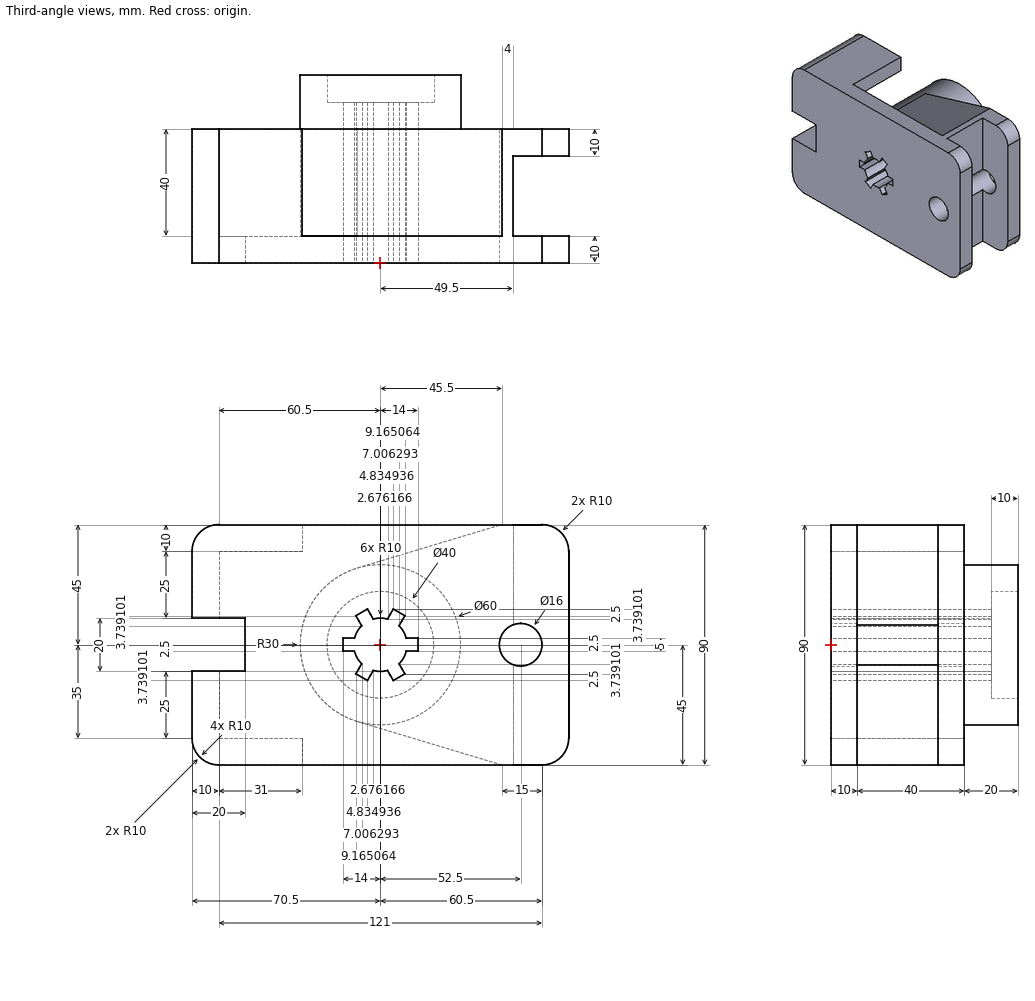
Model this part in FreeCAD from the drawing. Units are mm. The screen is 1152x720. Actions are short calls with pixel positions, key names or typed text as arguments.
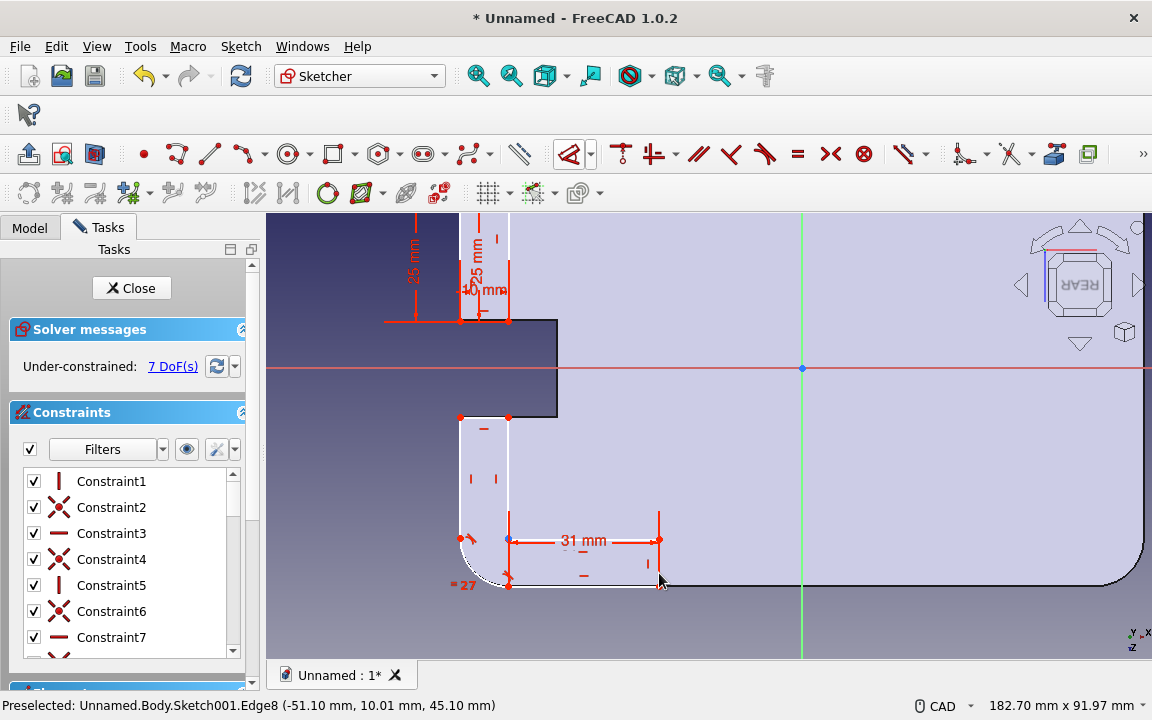
click(659, 573)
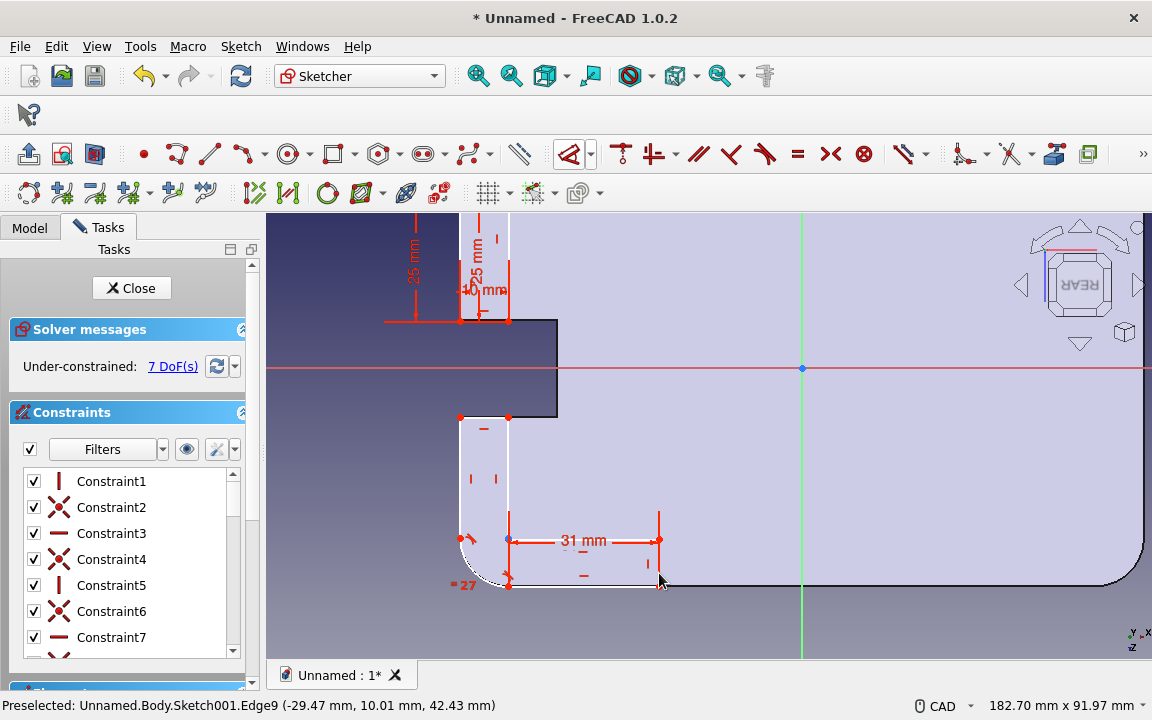
click(590, 154)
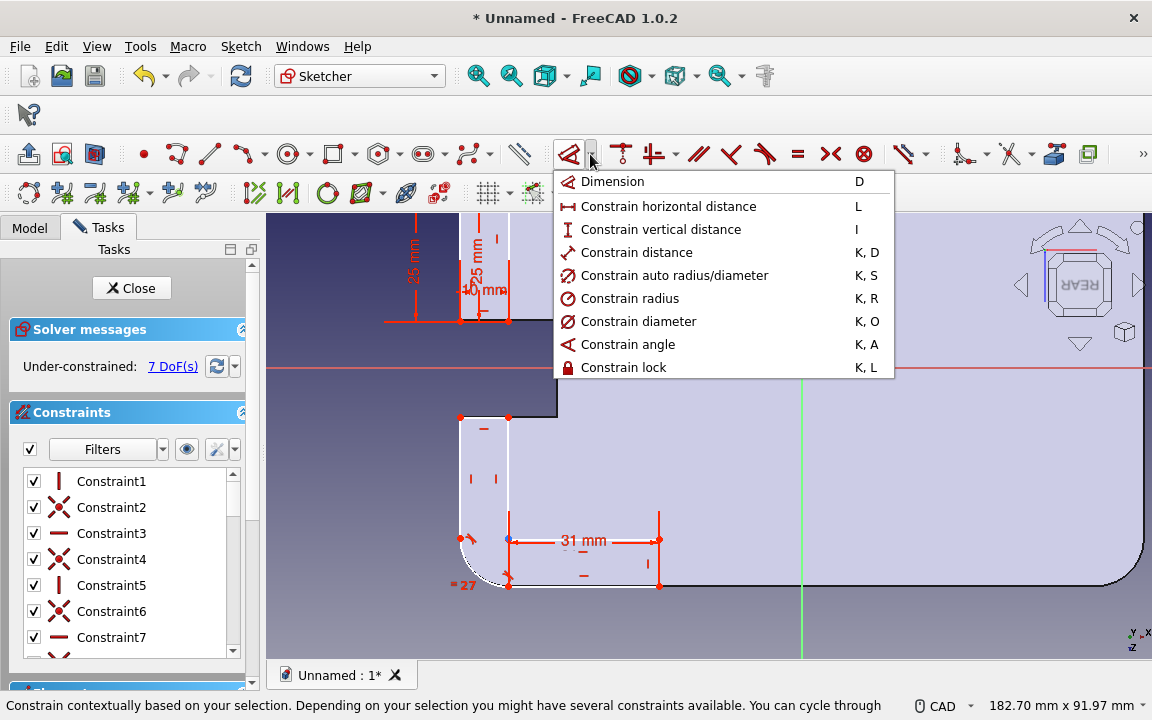
click(724, 230)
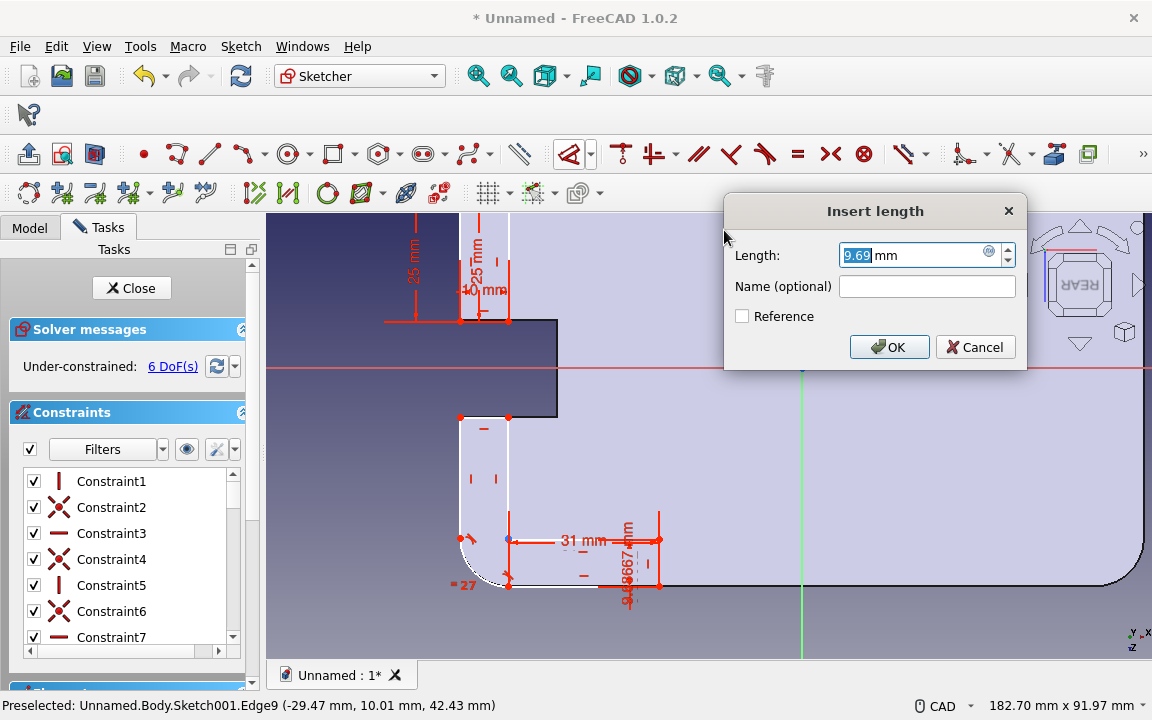
text(10)
key(Return)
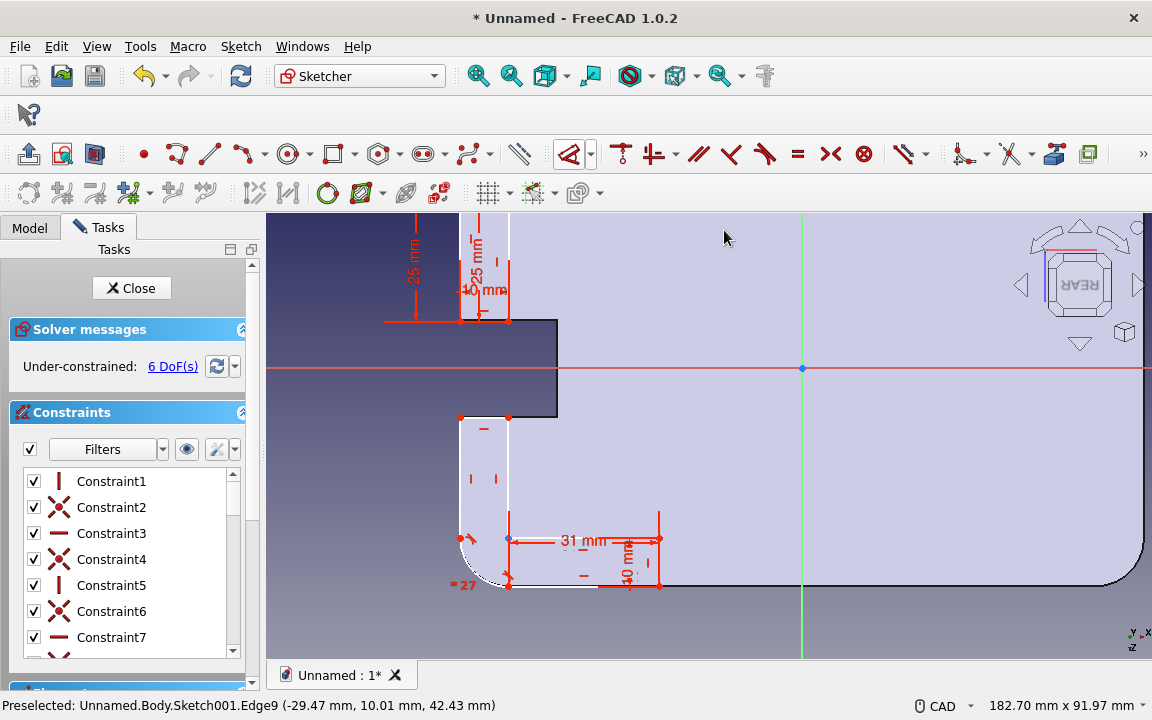
click(614, 538)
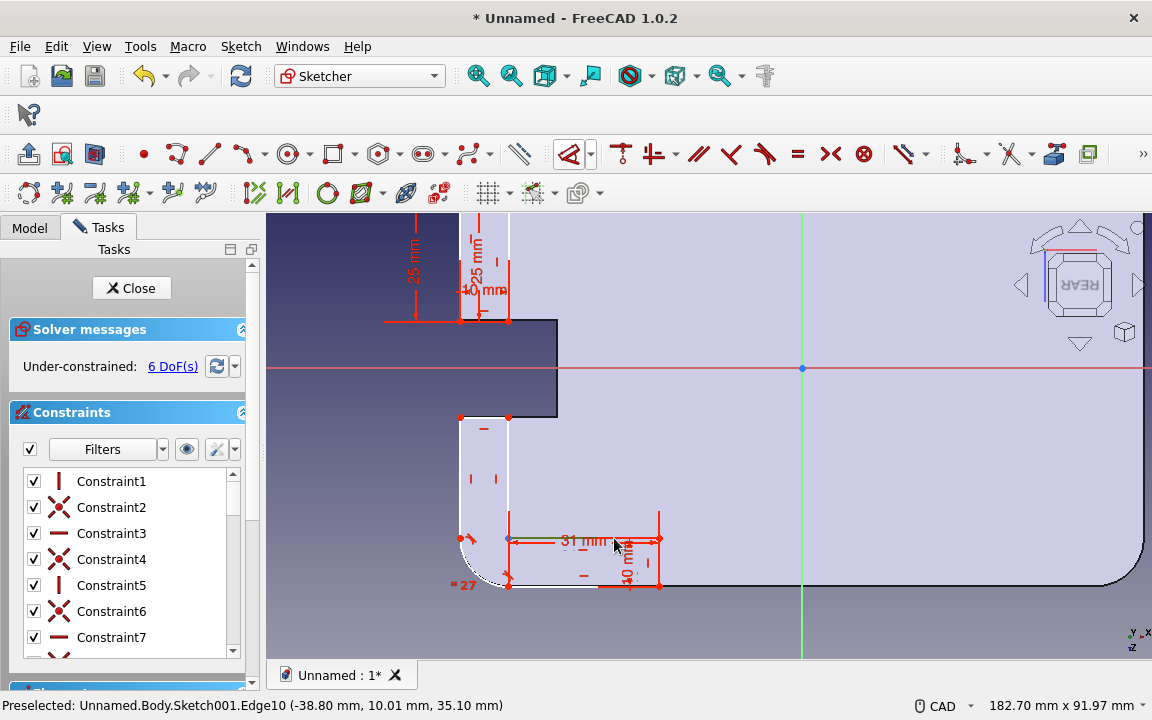
key(l)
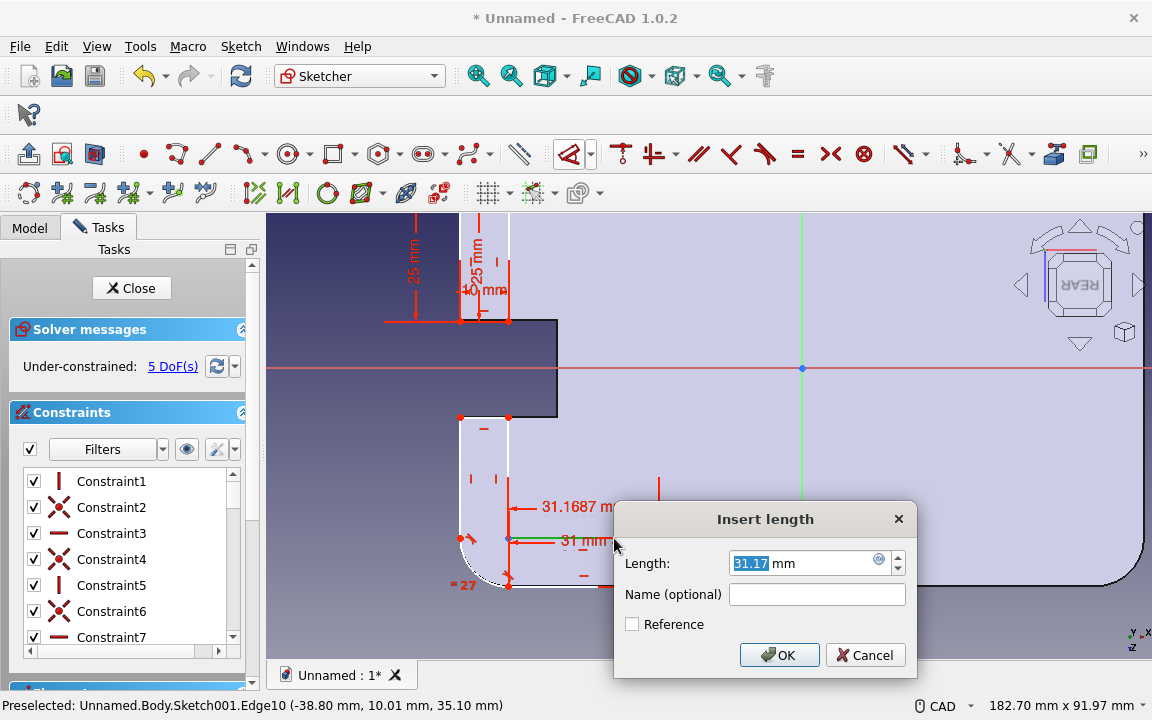
text(31)
key(Return)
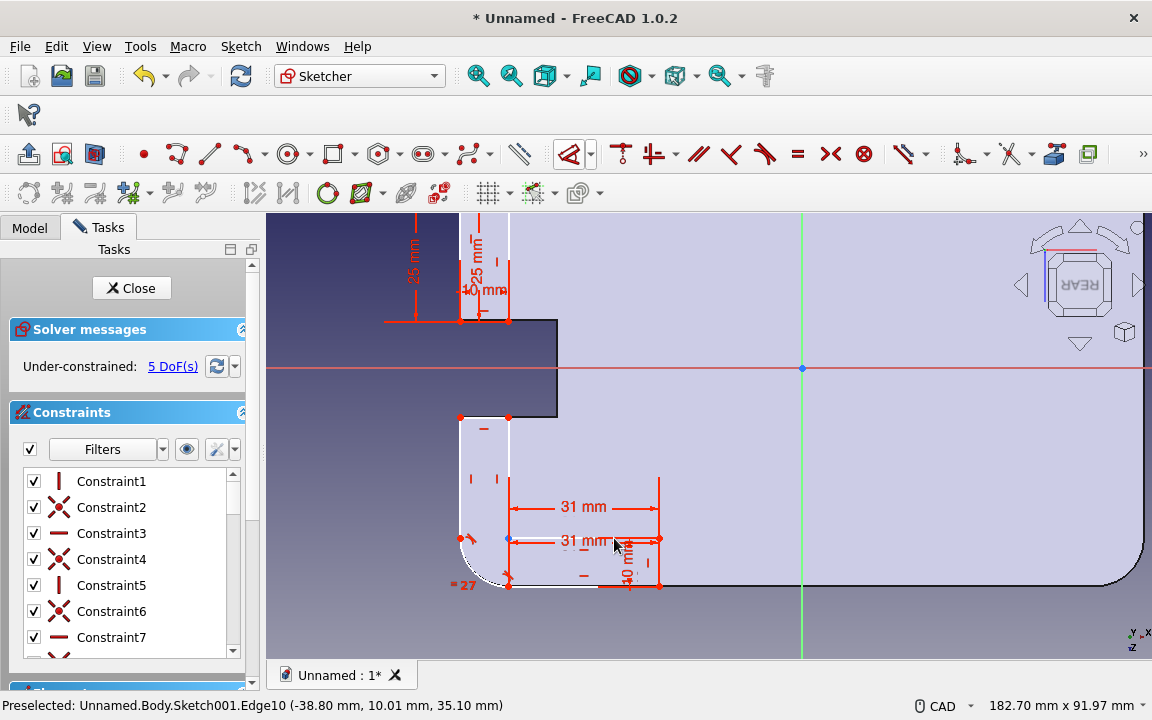
click(509, 502)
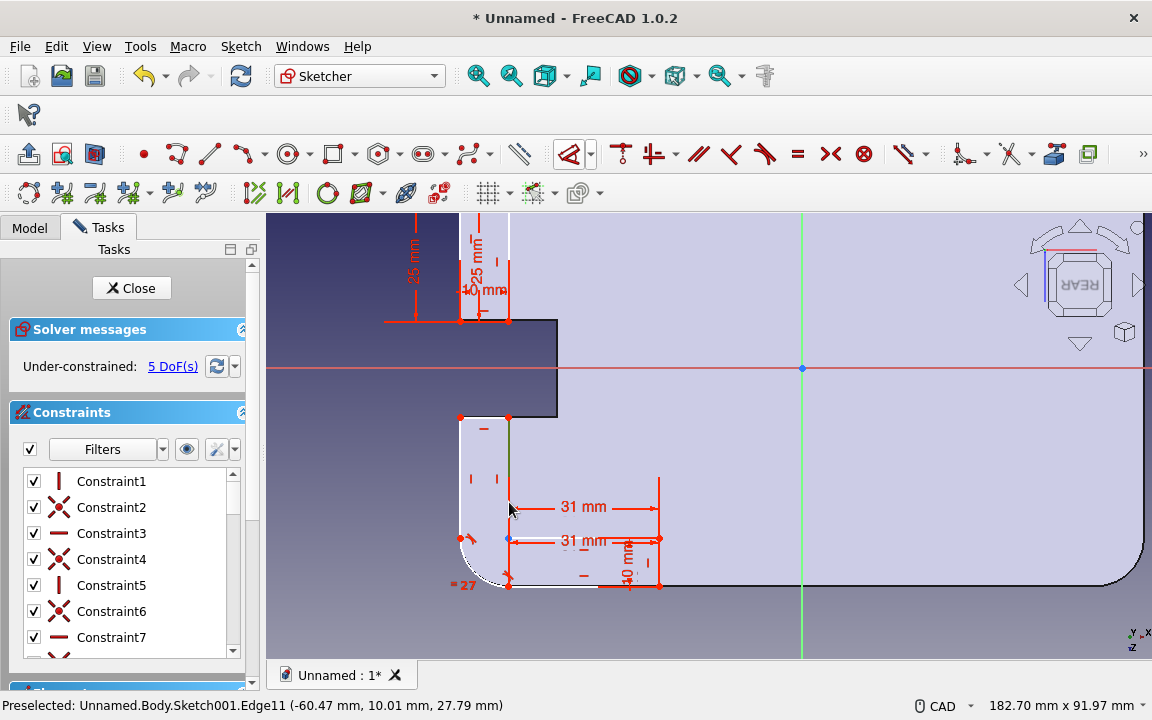
click(590, 154)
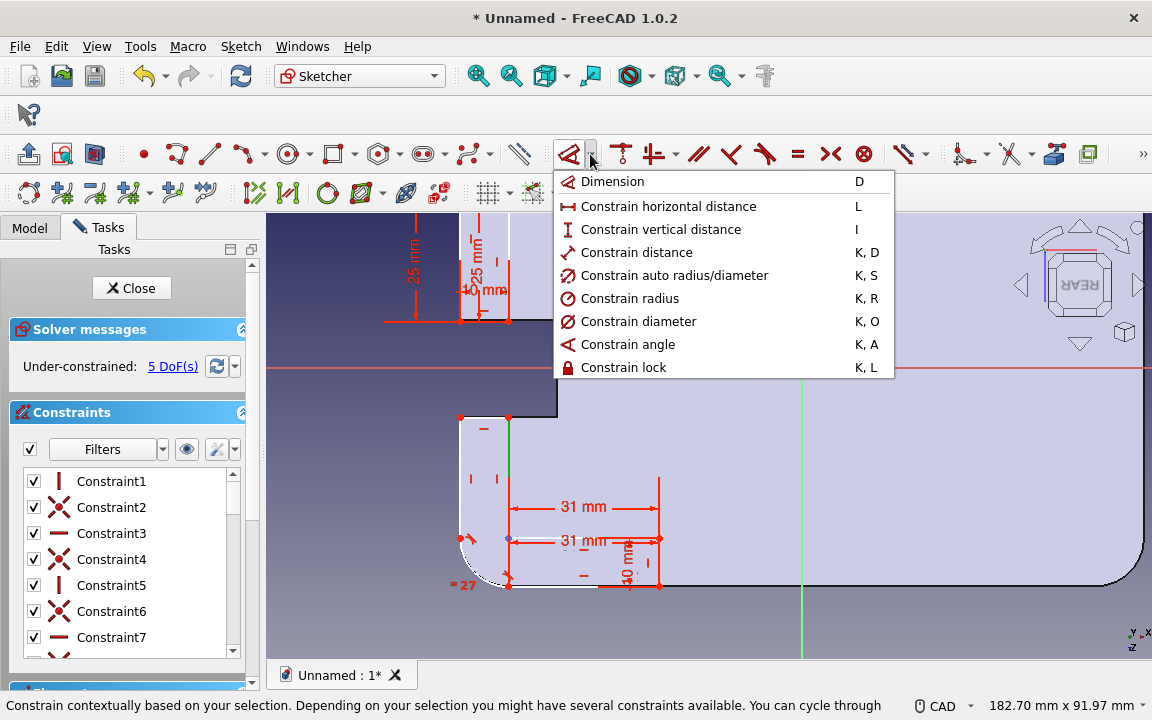
click(724, 230)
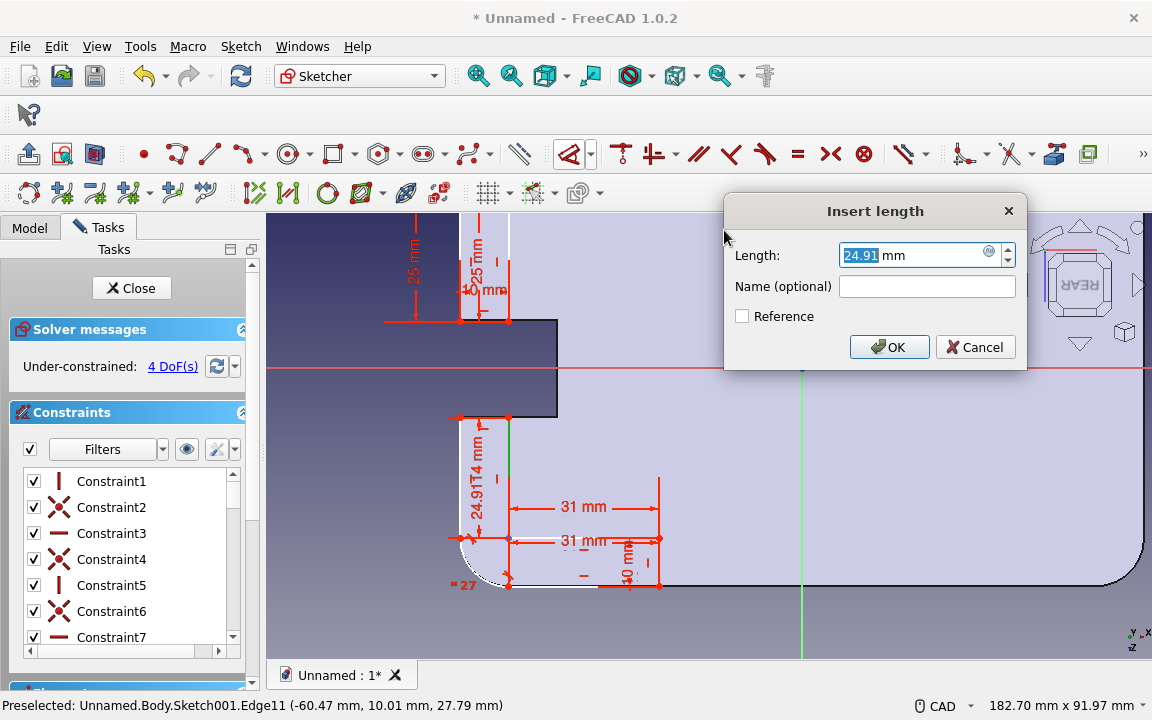
text(25)
key(Return)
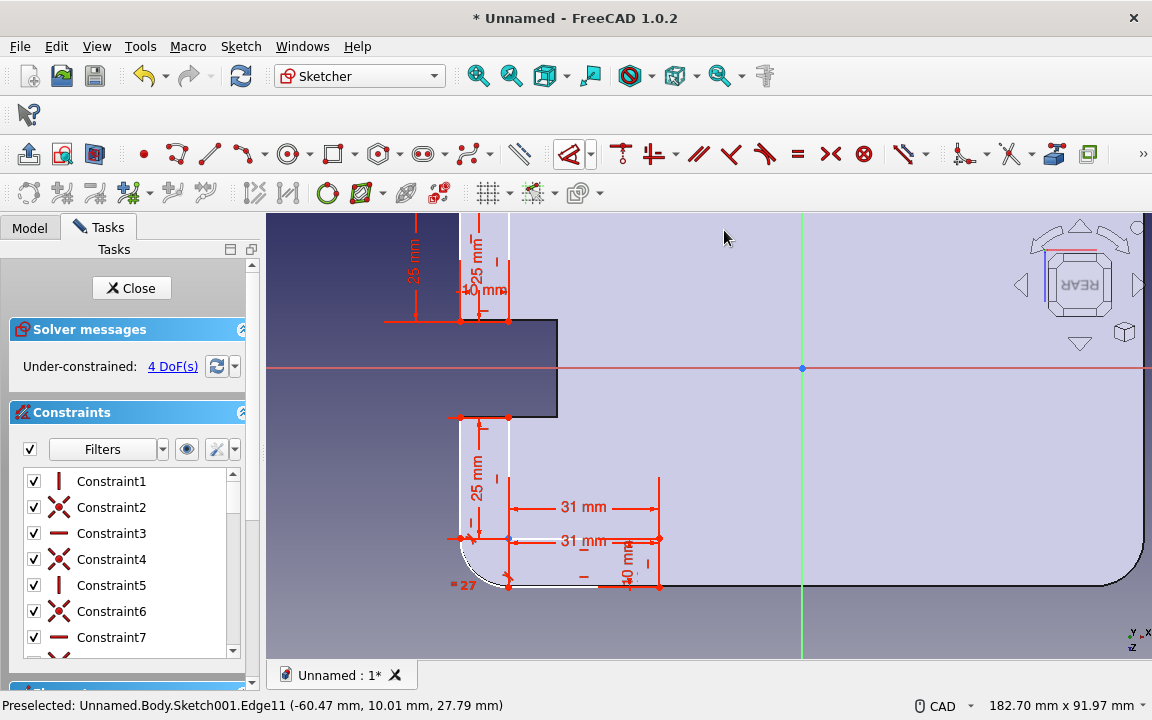
scroll(659, 574, down, 2)